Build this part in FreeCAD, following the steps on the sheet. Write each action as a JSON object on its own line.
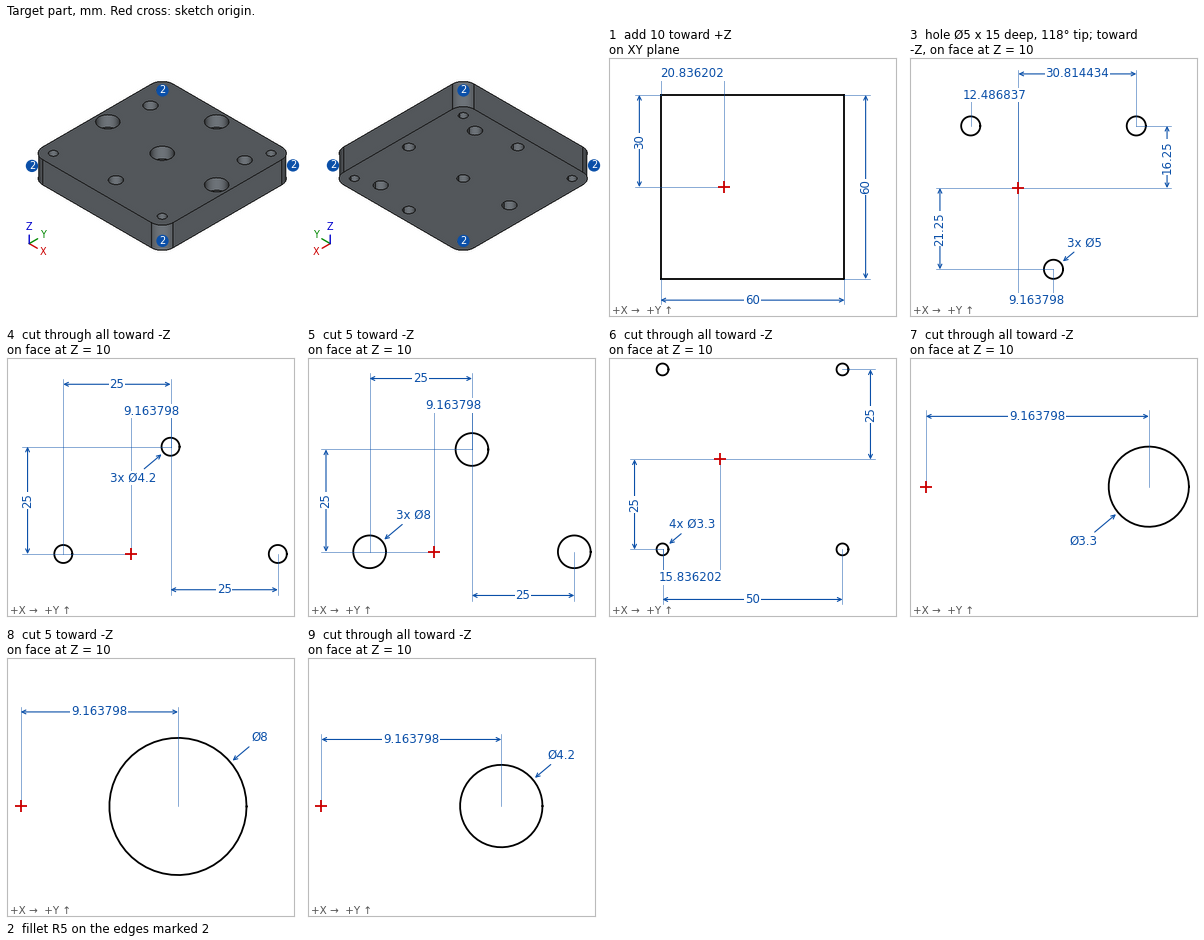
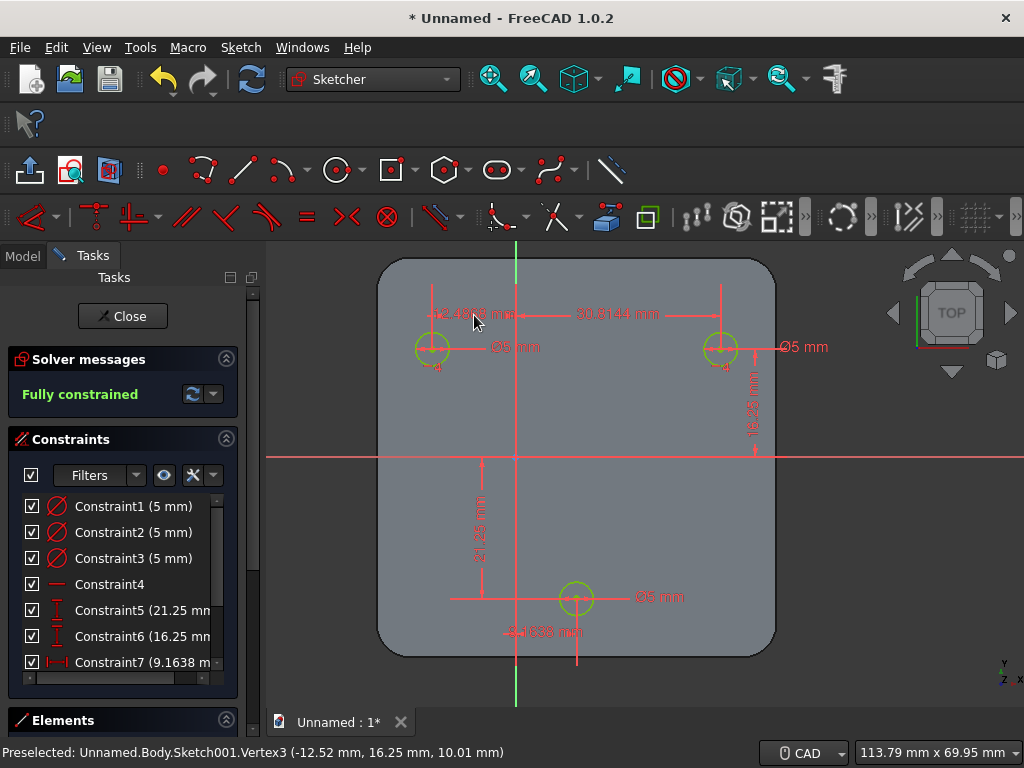
{"action": "left_click", "coordinate": [123, 316]}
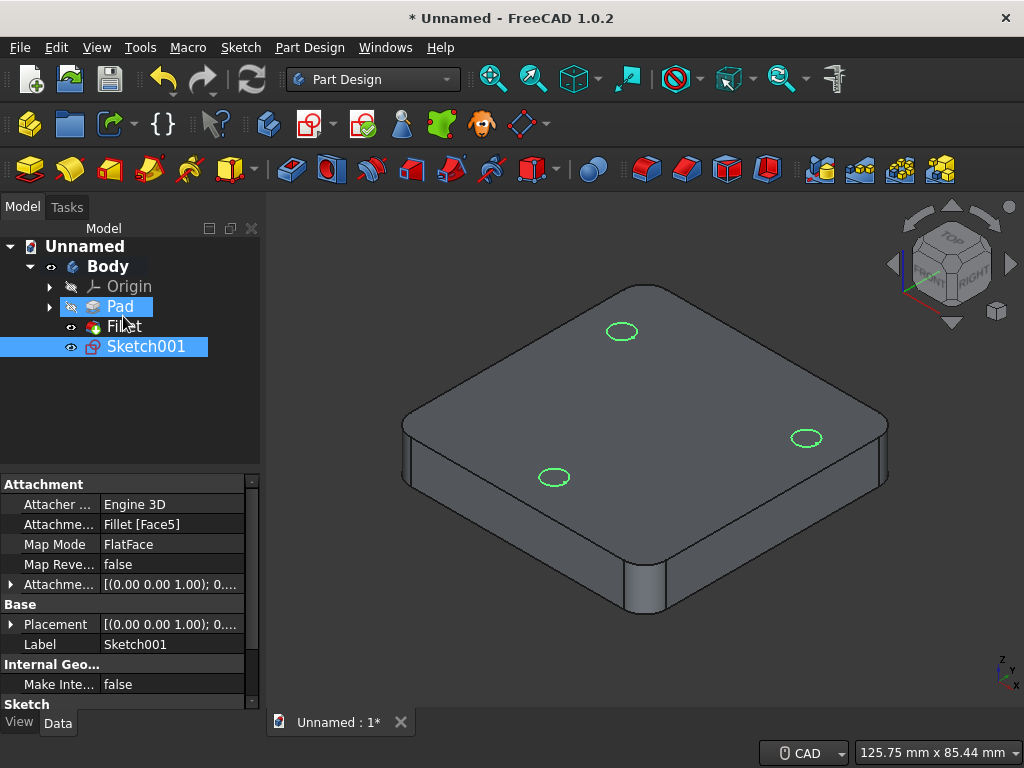
{"action": "left_click", "coordinate": [332, 170]}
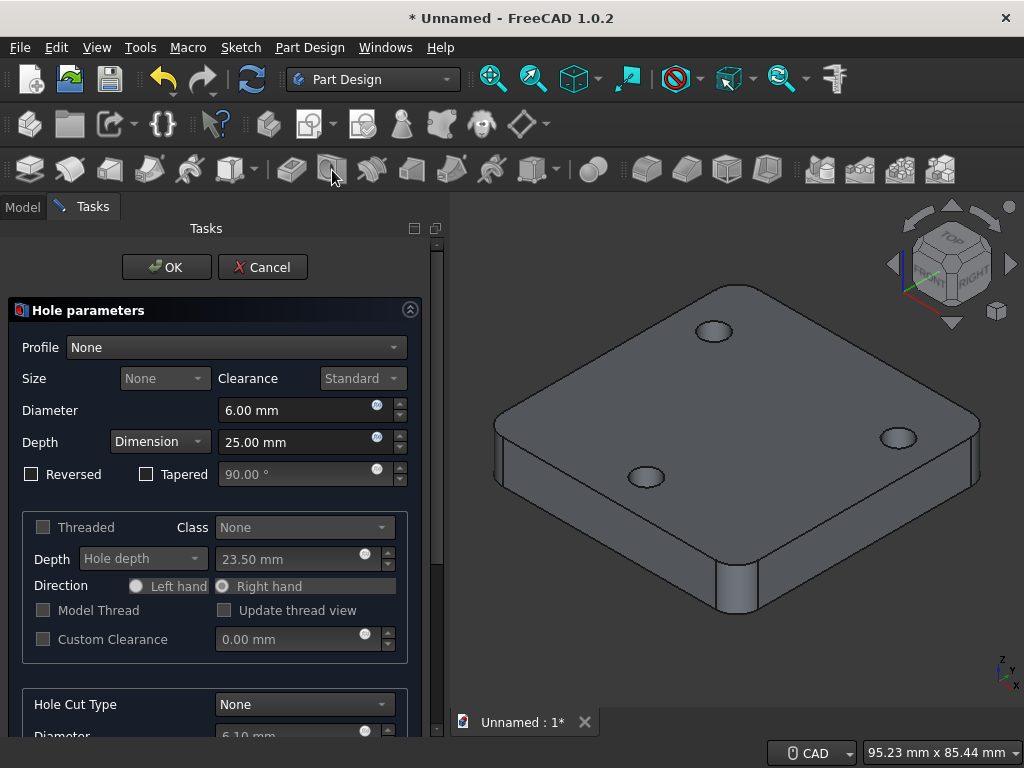
{"action": "triple_click", "coordinate": [305, 410]}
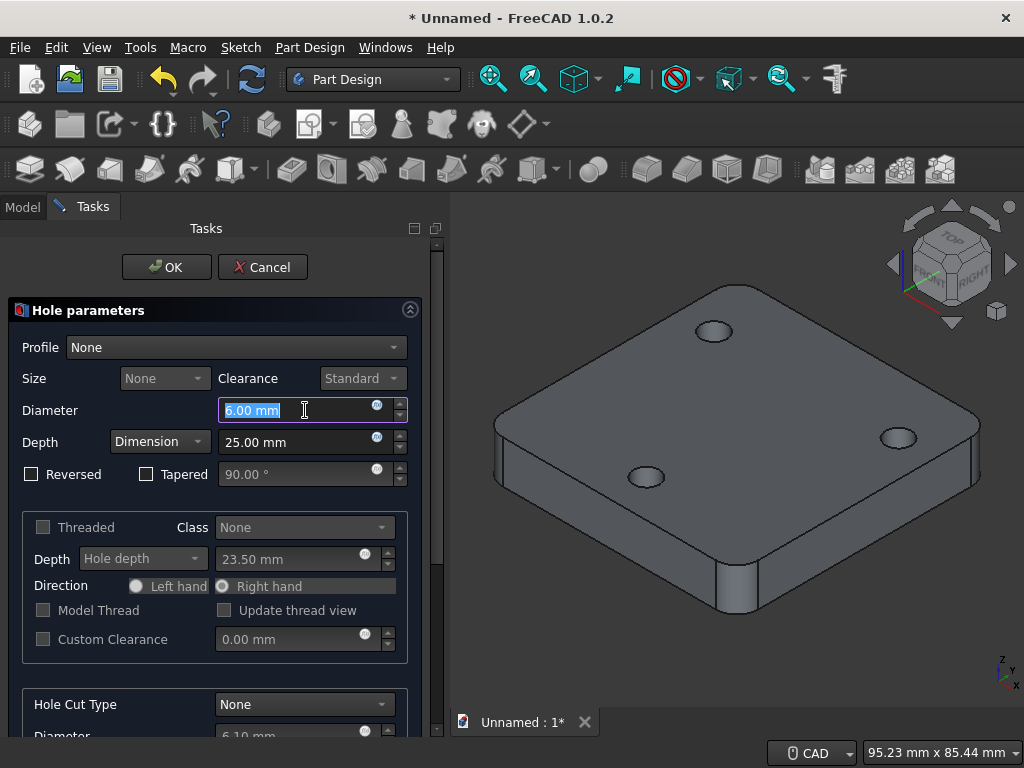
{"action": "type", "text": "5"}
{"action": "key", "text": "Tab"}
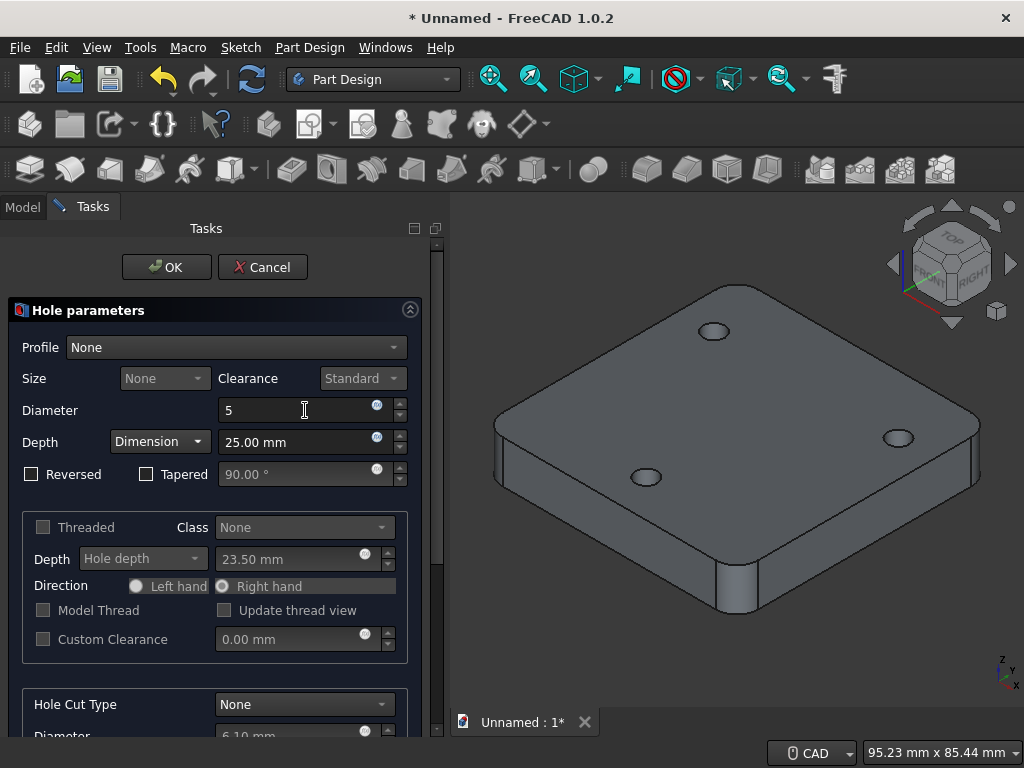
{"action": "triple_click", "coordinate": [305, 442]}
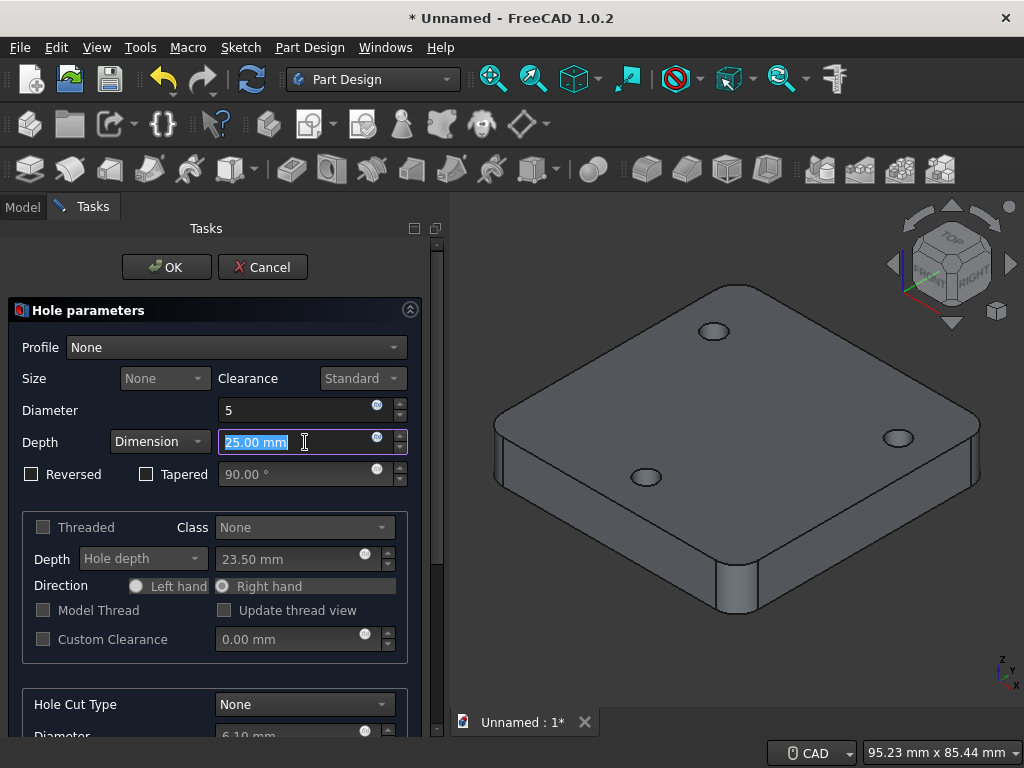
{"action": "type", "text": "15"}
{"action": "key", "text": "Tab"}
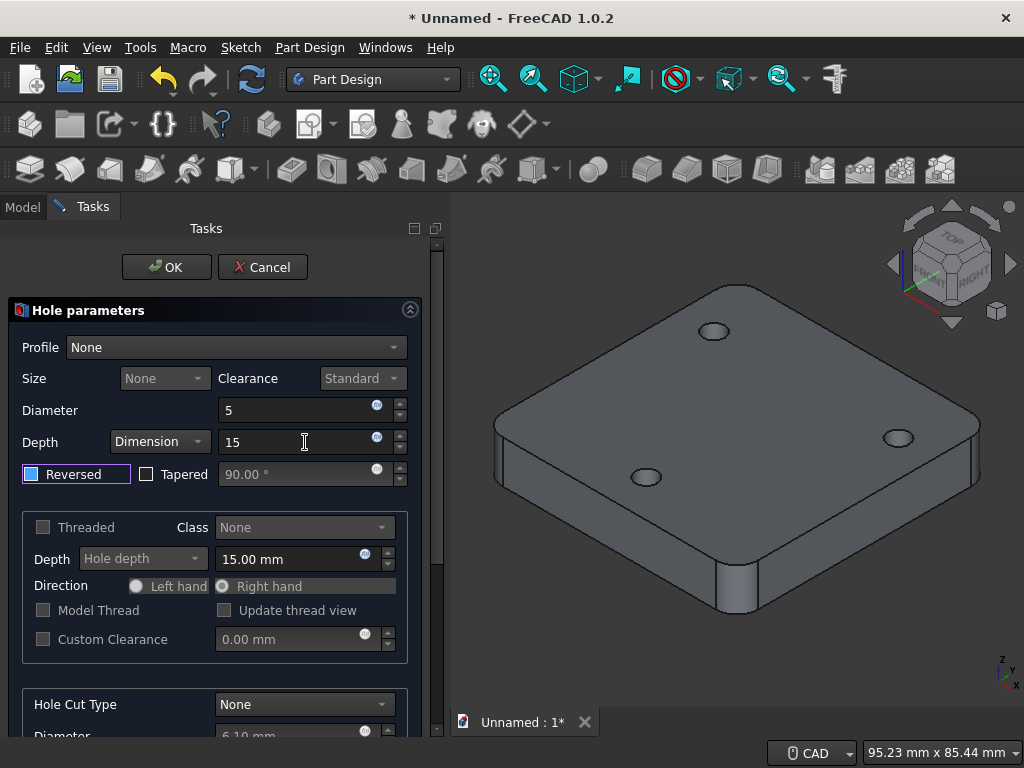
{"action": "left_click", "coordinate": [167, 267]}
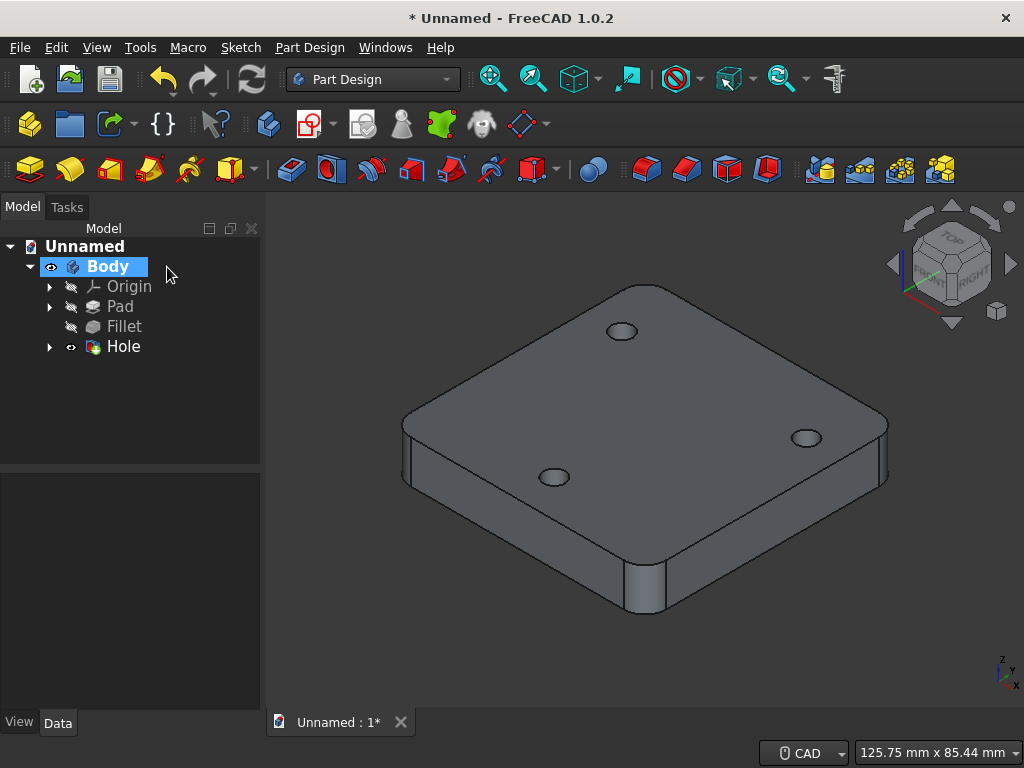
{"action": "left_click", "coordinate": [682, 403]}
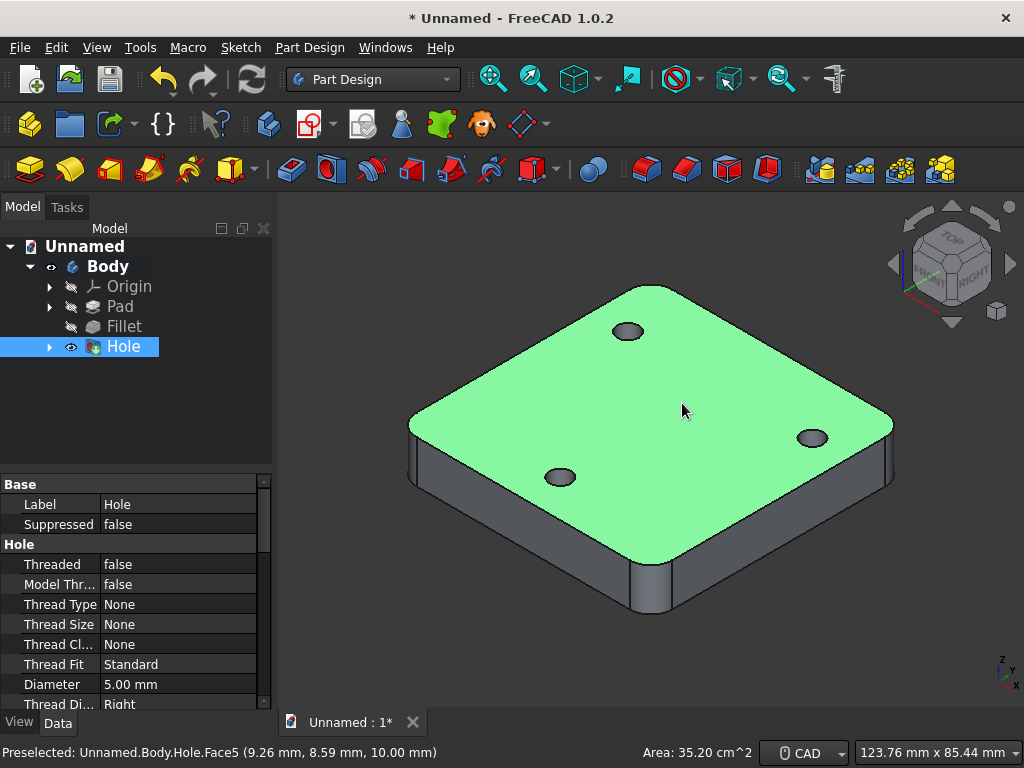
{"action": "left_click", "coordinate": [310, 124]}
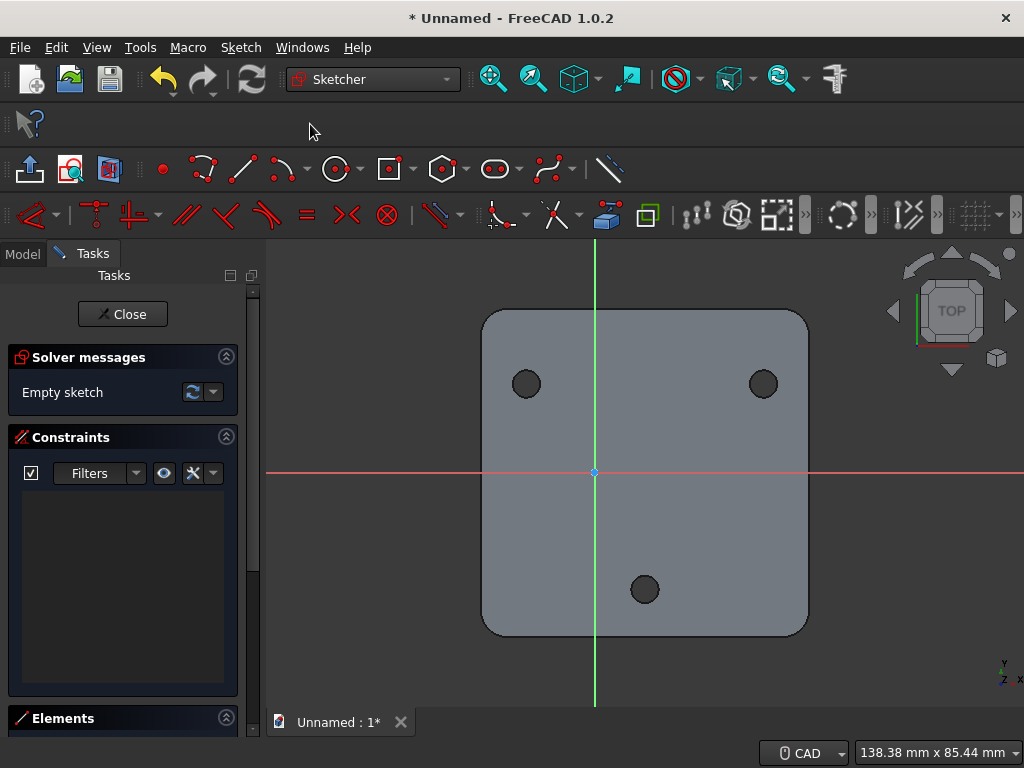
{"action": "left_click", "coordinate": [336, 170]}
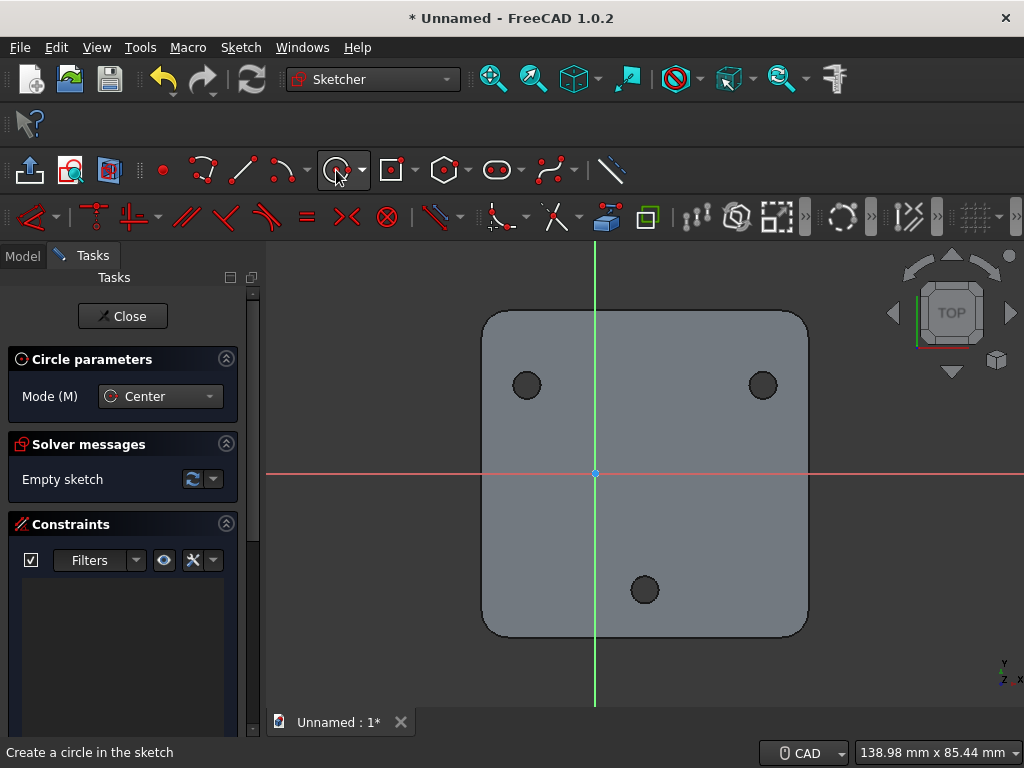
{"action": "scroll", "coordinate": [645, 338], "scroll_direction": "up", "scroll_amount": 4}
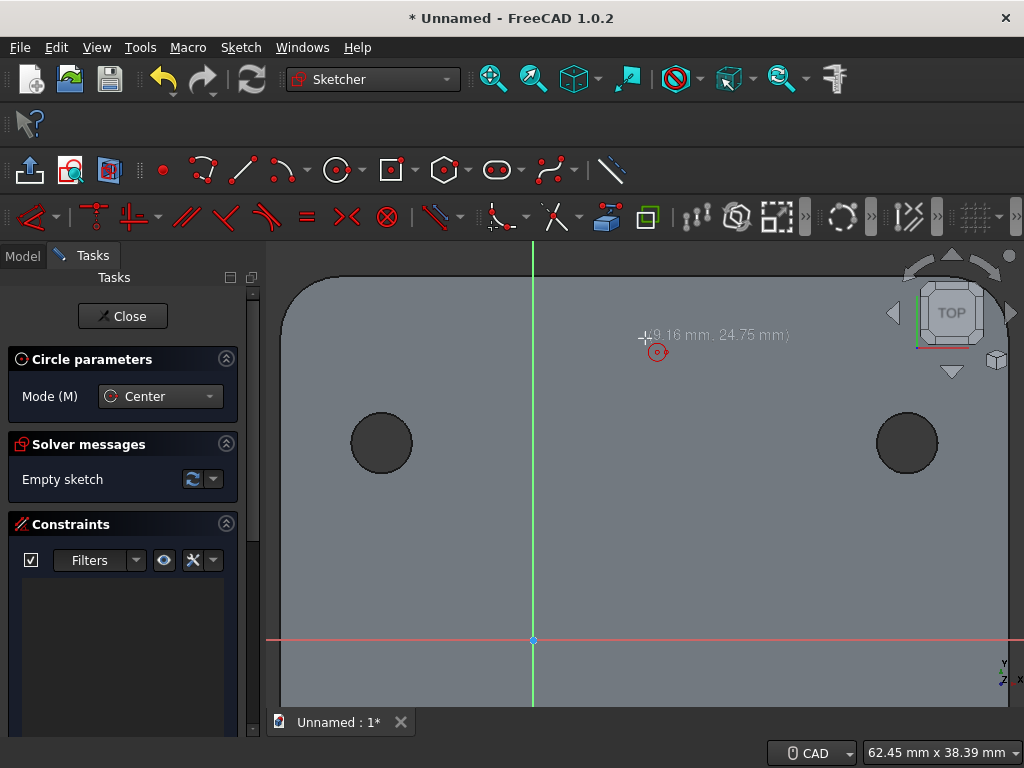
{"action": "left_click", "coordinate": [644, 337]}
{"action": "mouse_move", "coordinate": [662, 319]}